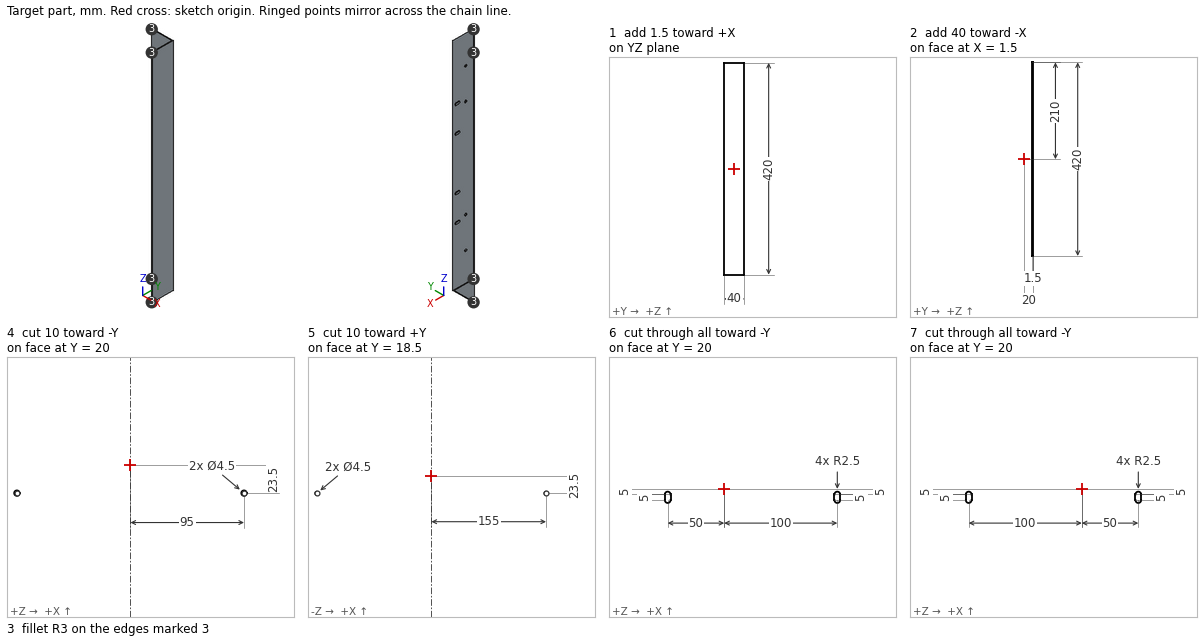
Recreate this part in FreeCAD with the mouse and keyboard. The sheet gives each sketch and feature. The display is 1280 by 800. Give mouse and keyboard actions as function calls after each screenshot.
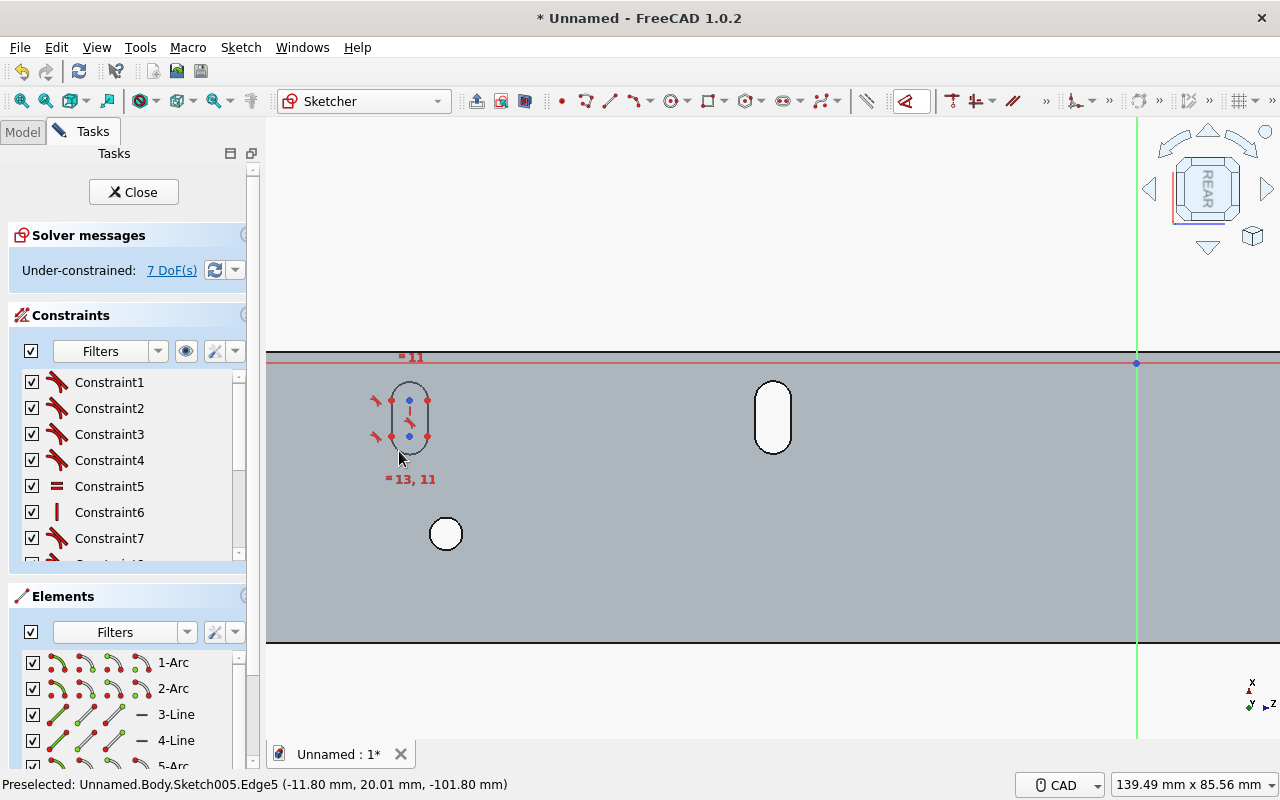
scroll(400, 452, down, 3)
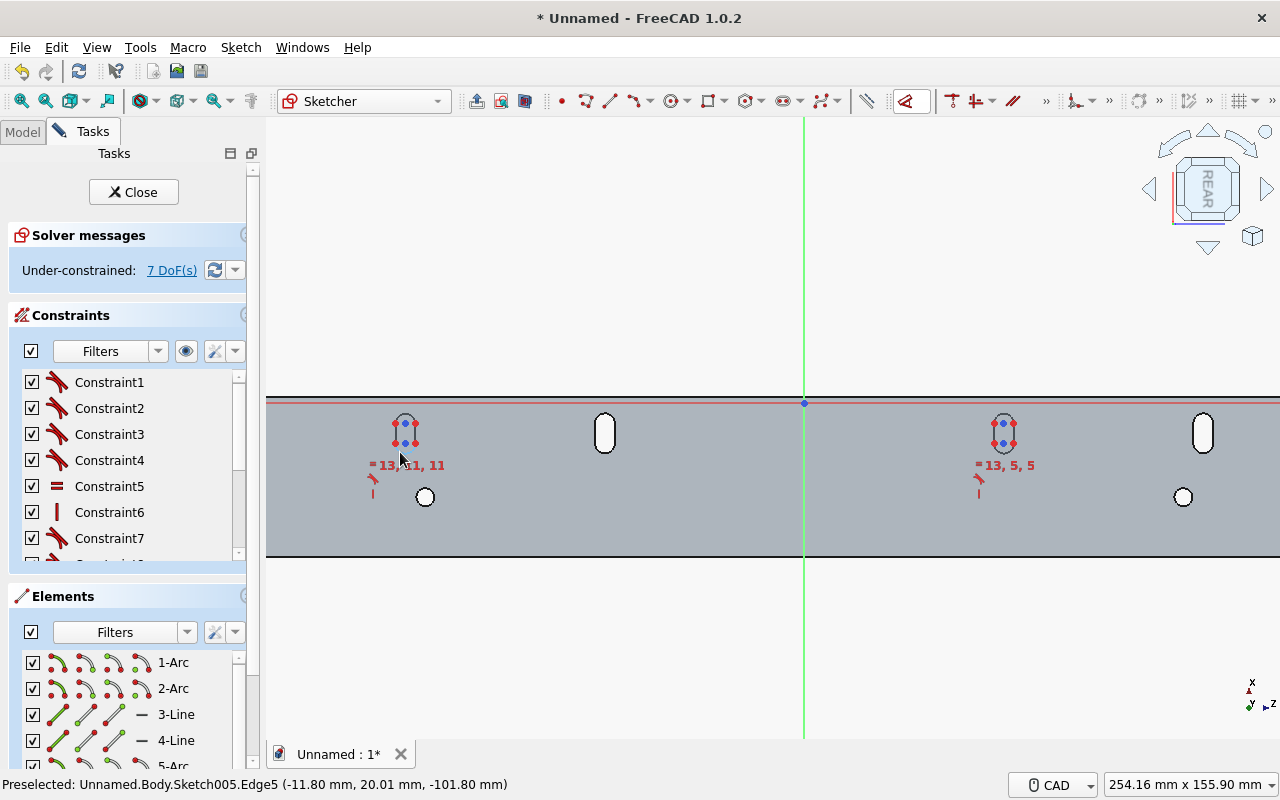
scroll(998, 452, up, 7)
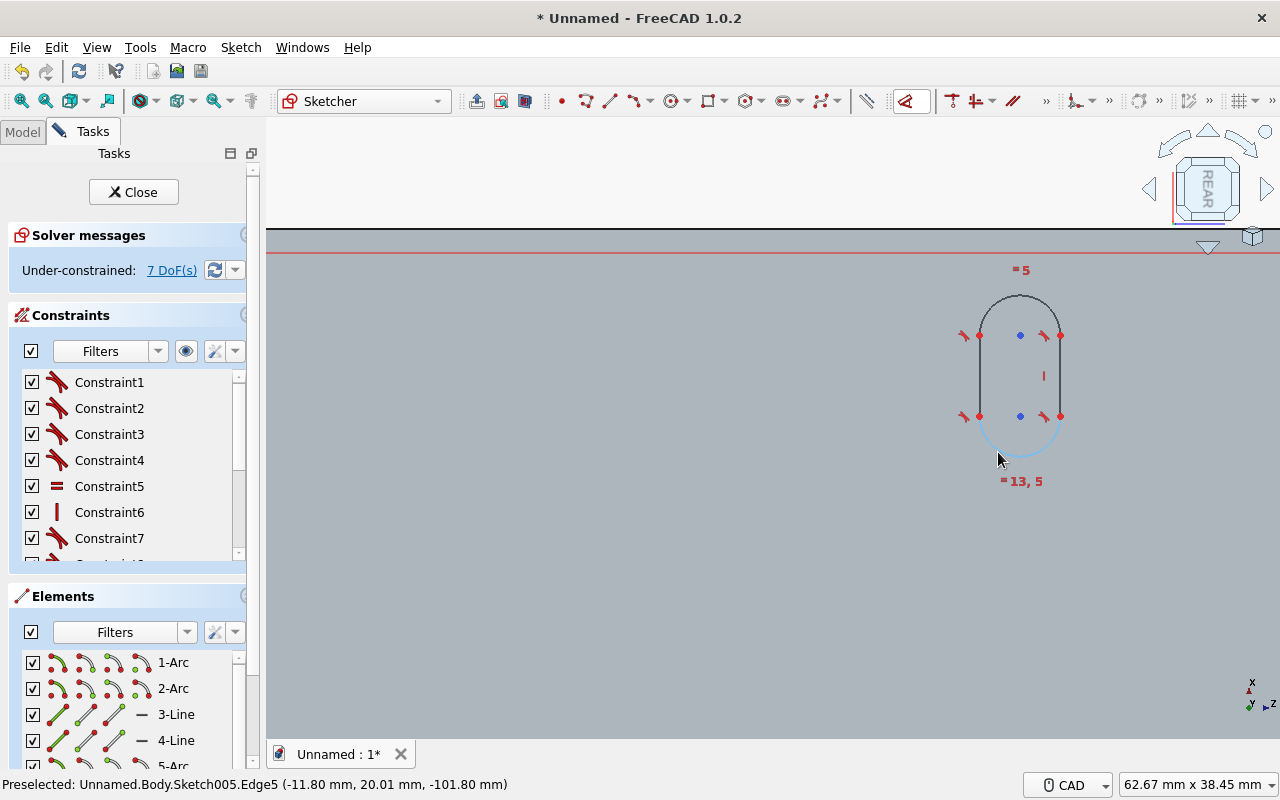
click(996, 449)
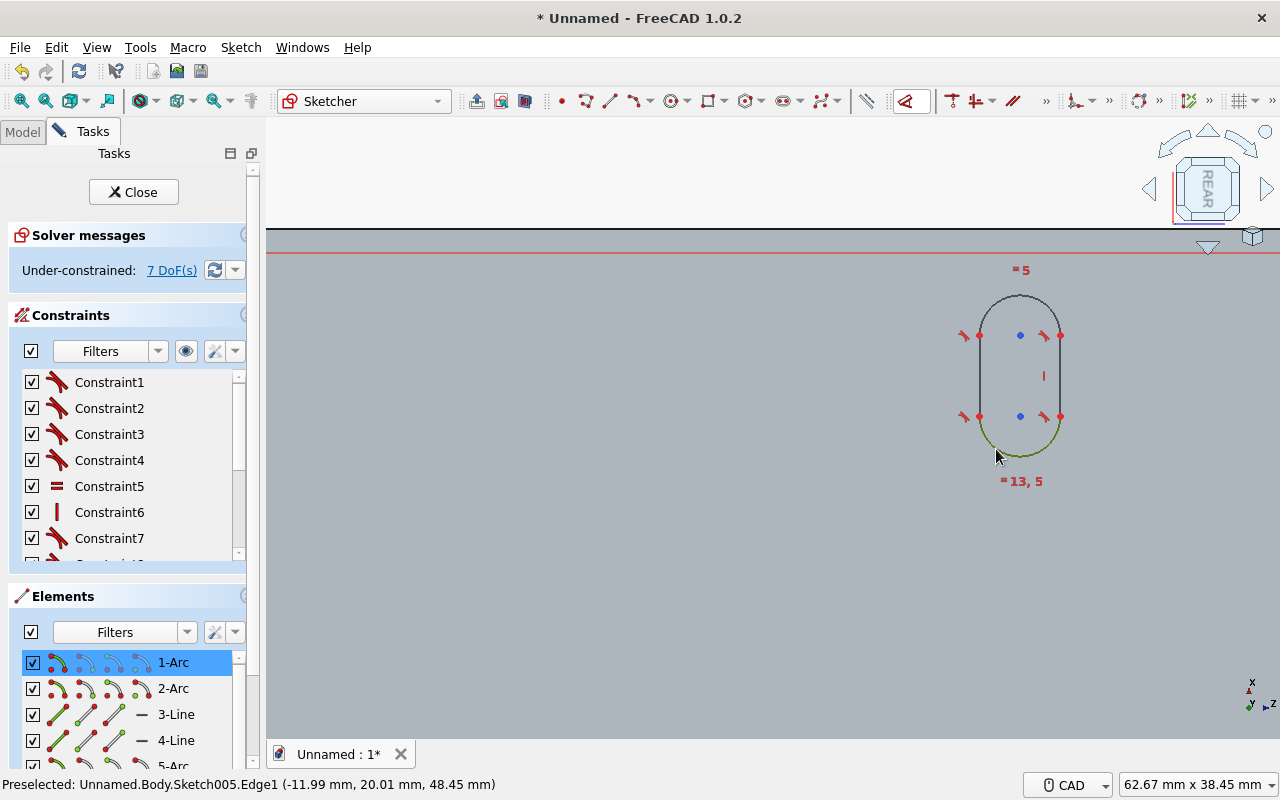
click(924, 102)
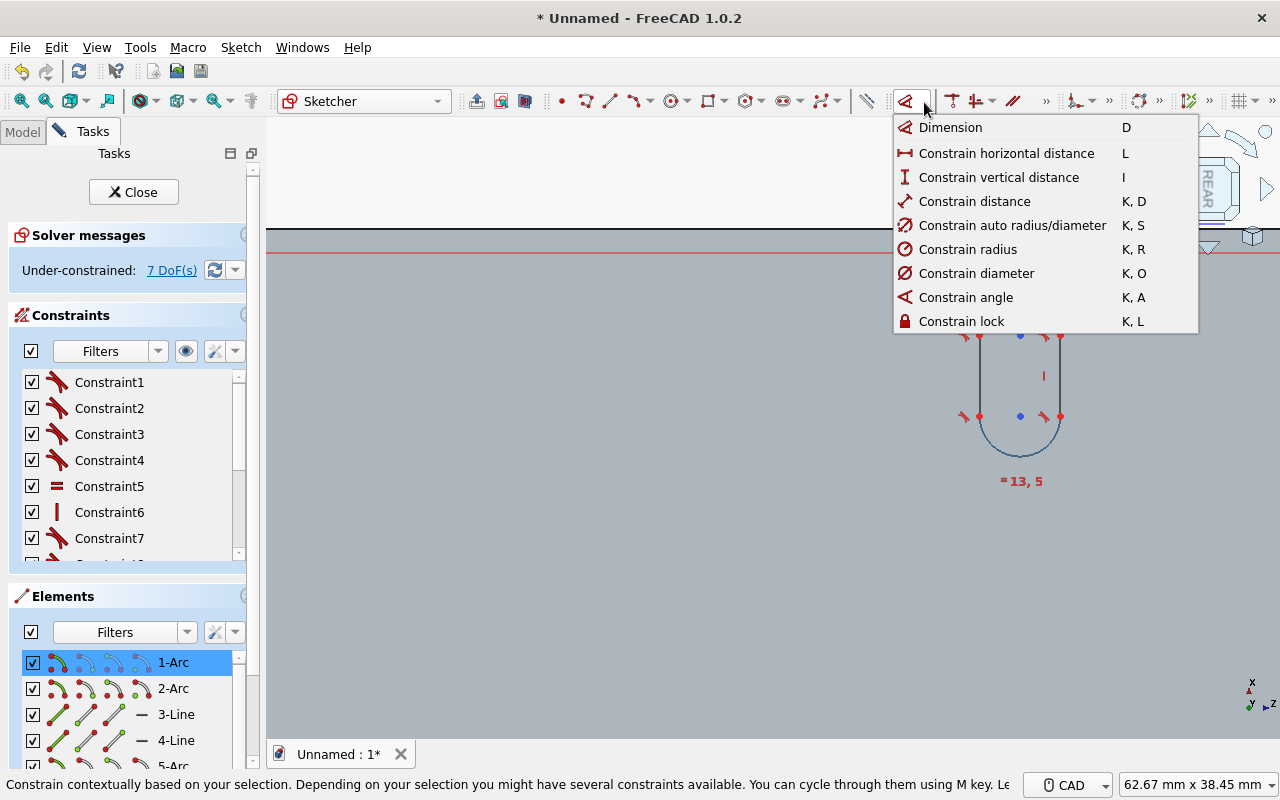
click(1046, 249)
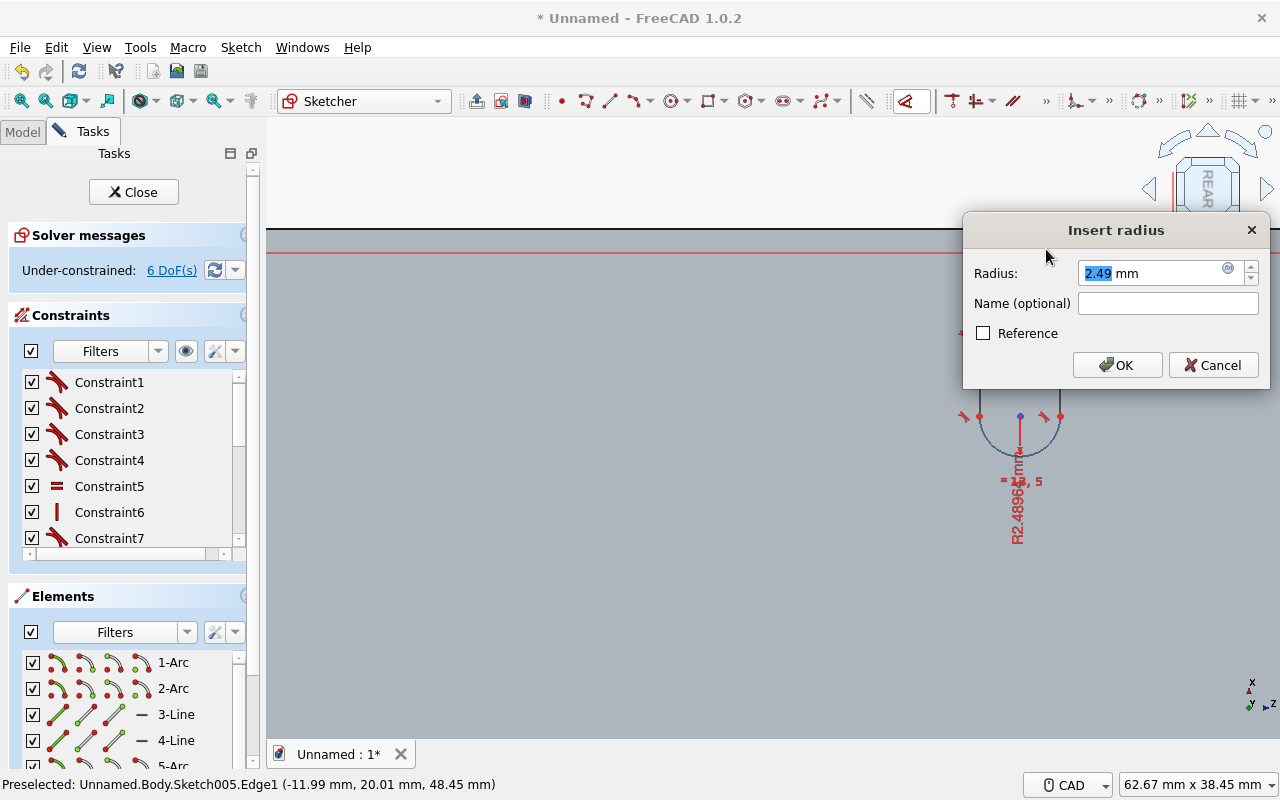
text(2.5)
key(Return)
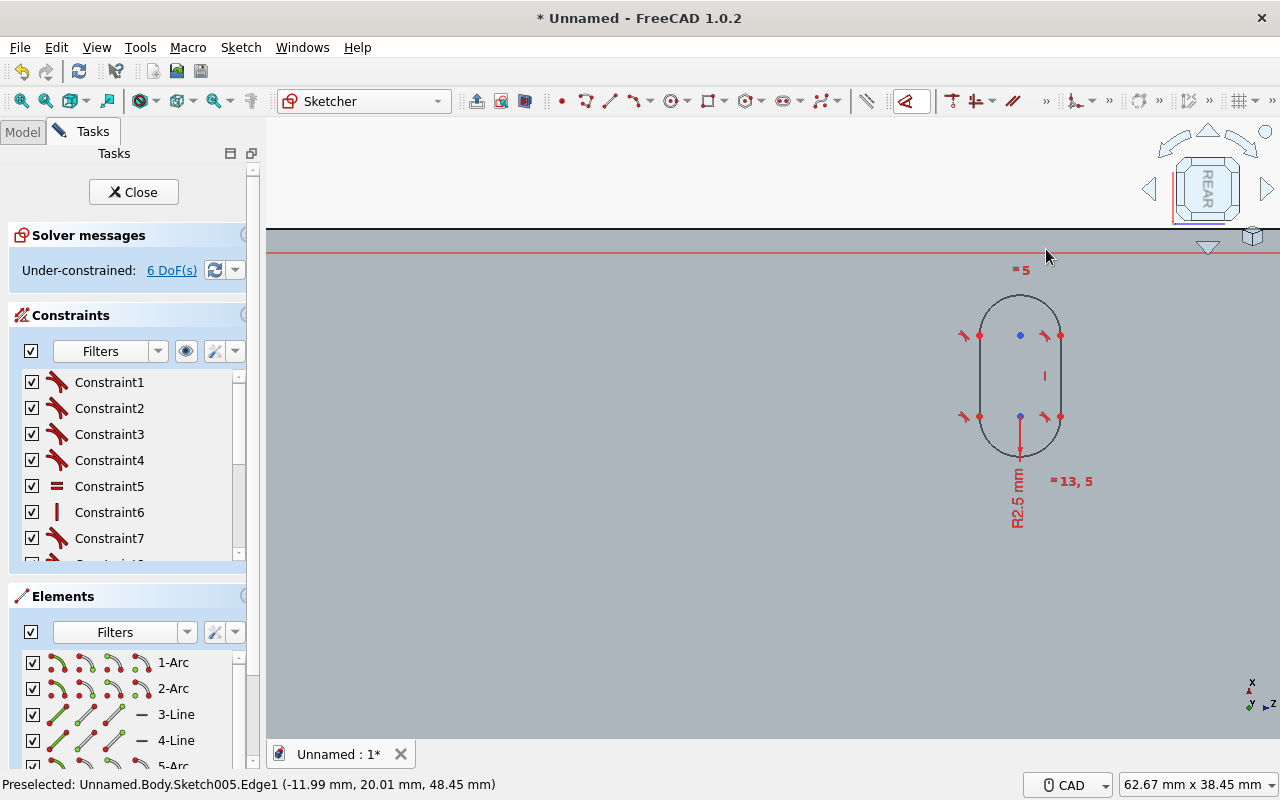
click(980, 392)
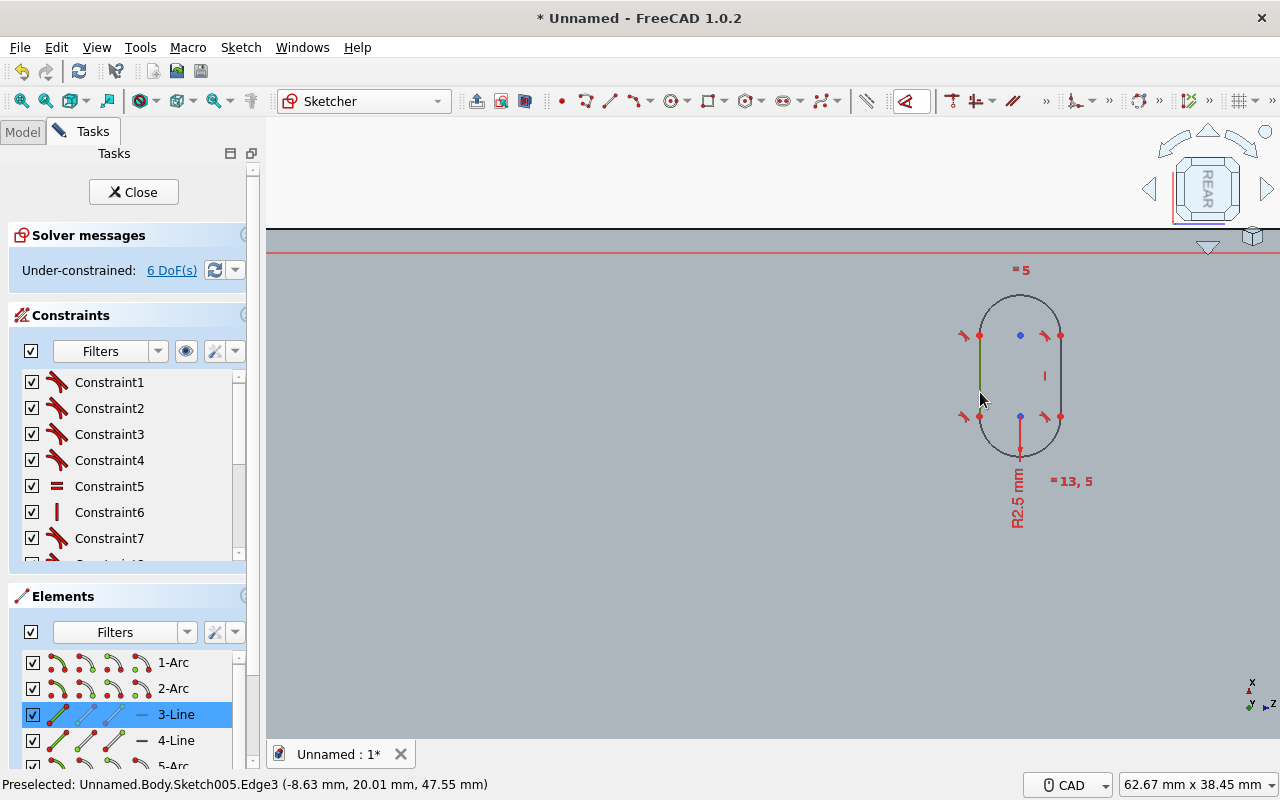
click(924, 102)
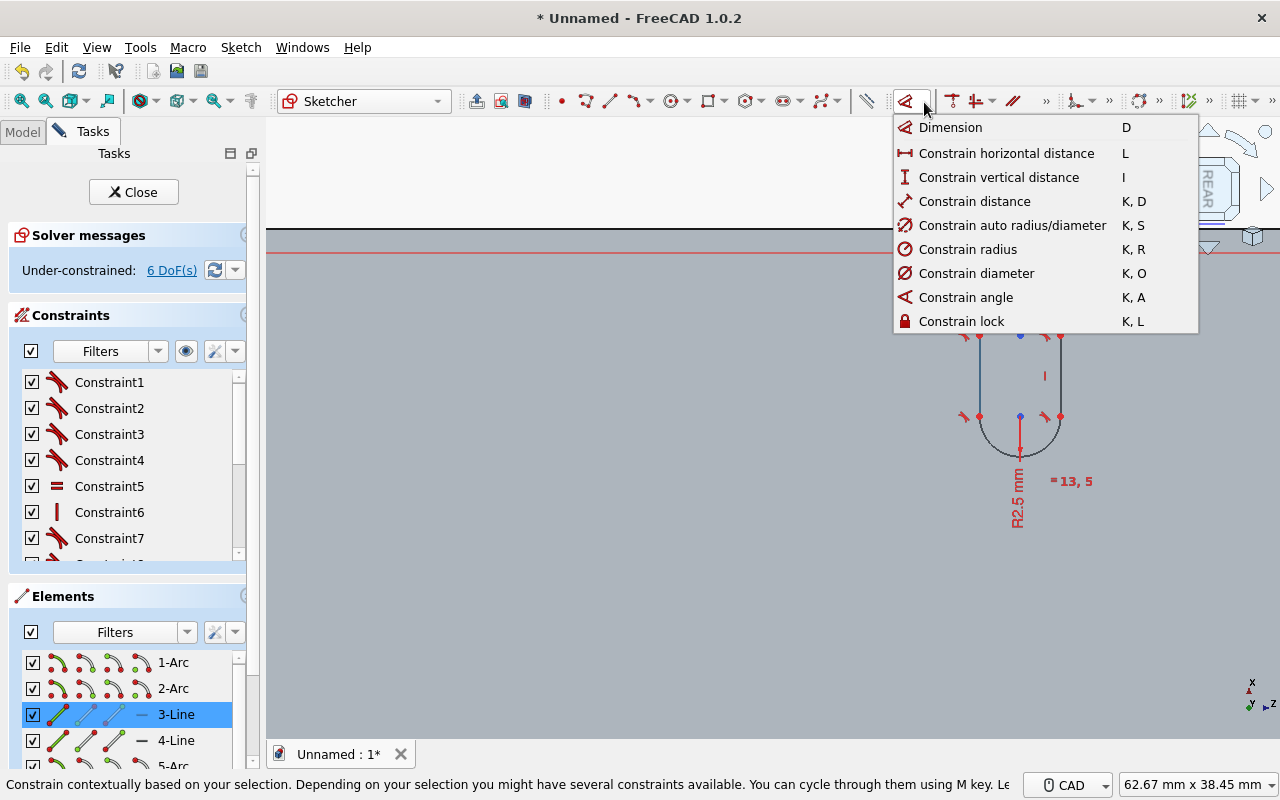
click(1046, 177)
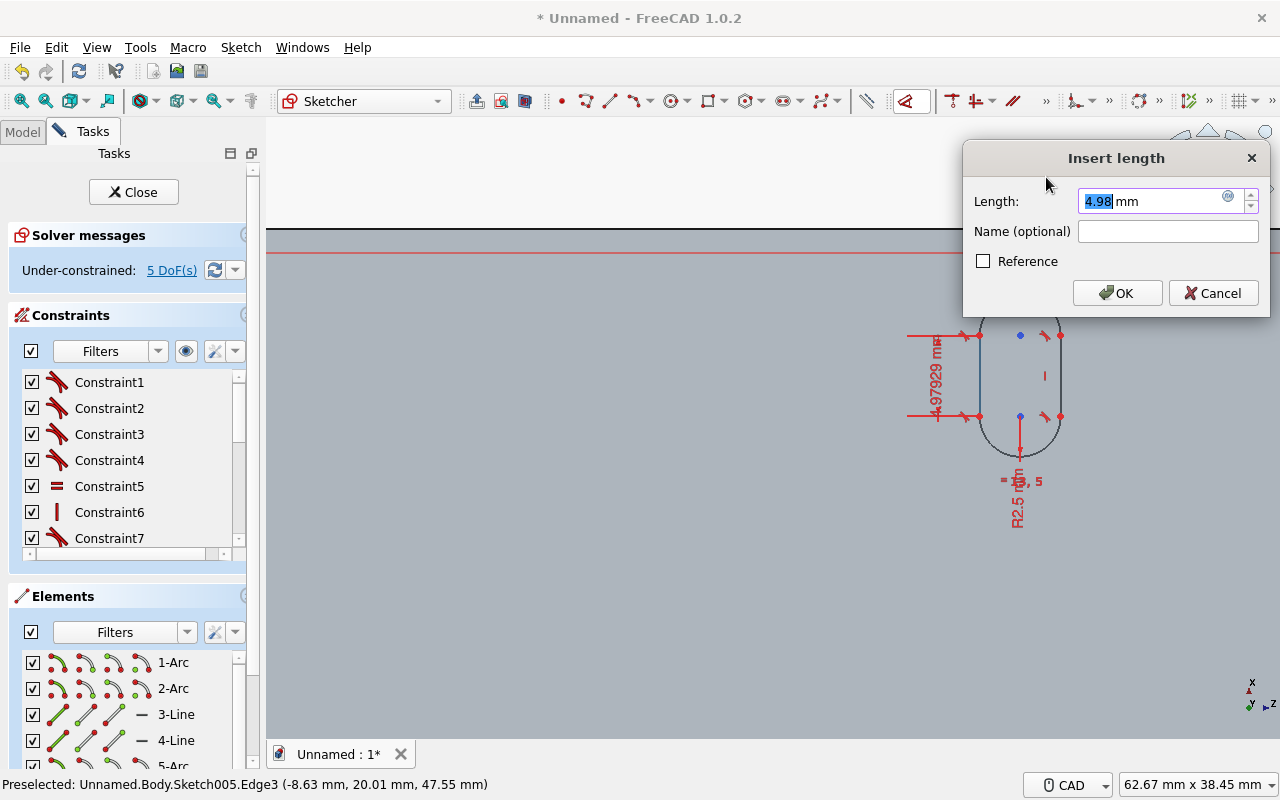
text(5)
key(Return)